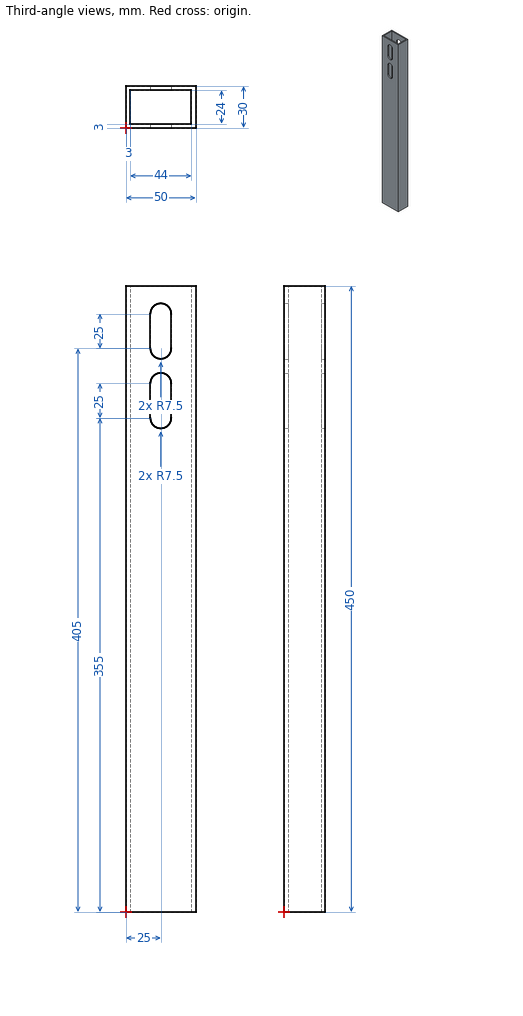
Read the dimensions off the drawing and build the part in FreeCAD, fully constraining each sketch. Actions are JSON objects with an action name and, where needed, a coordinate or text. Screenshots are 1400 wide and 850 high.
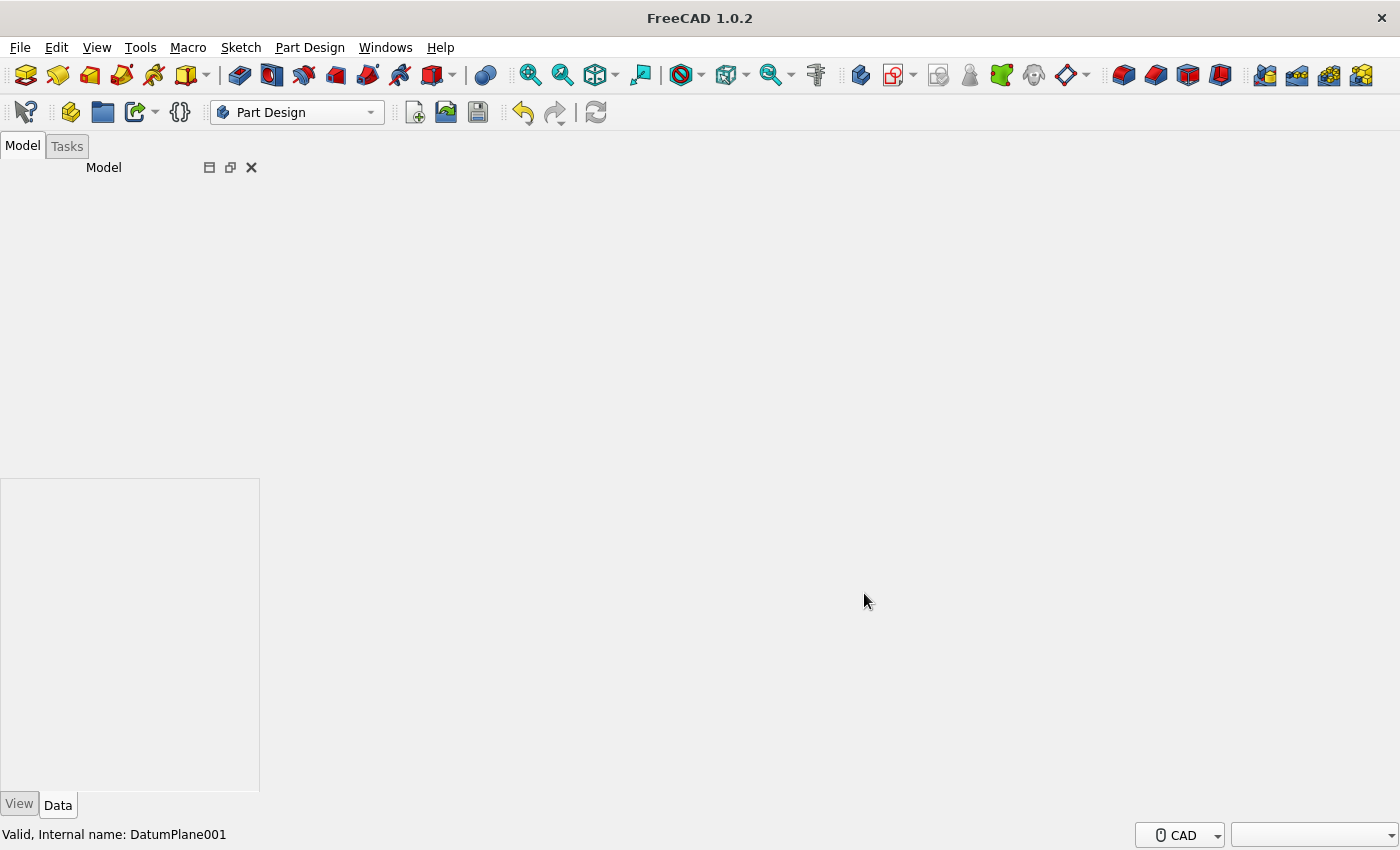
{"action": "left_click", "coordinate": [414, 112]}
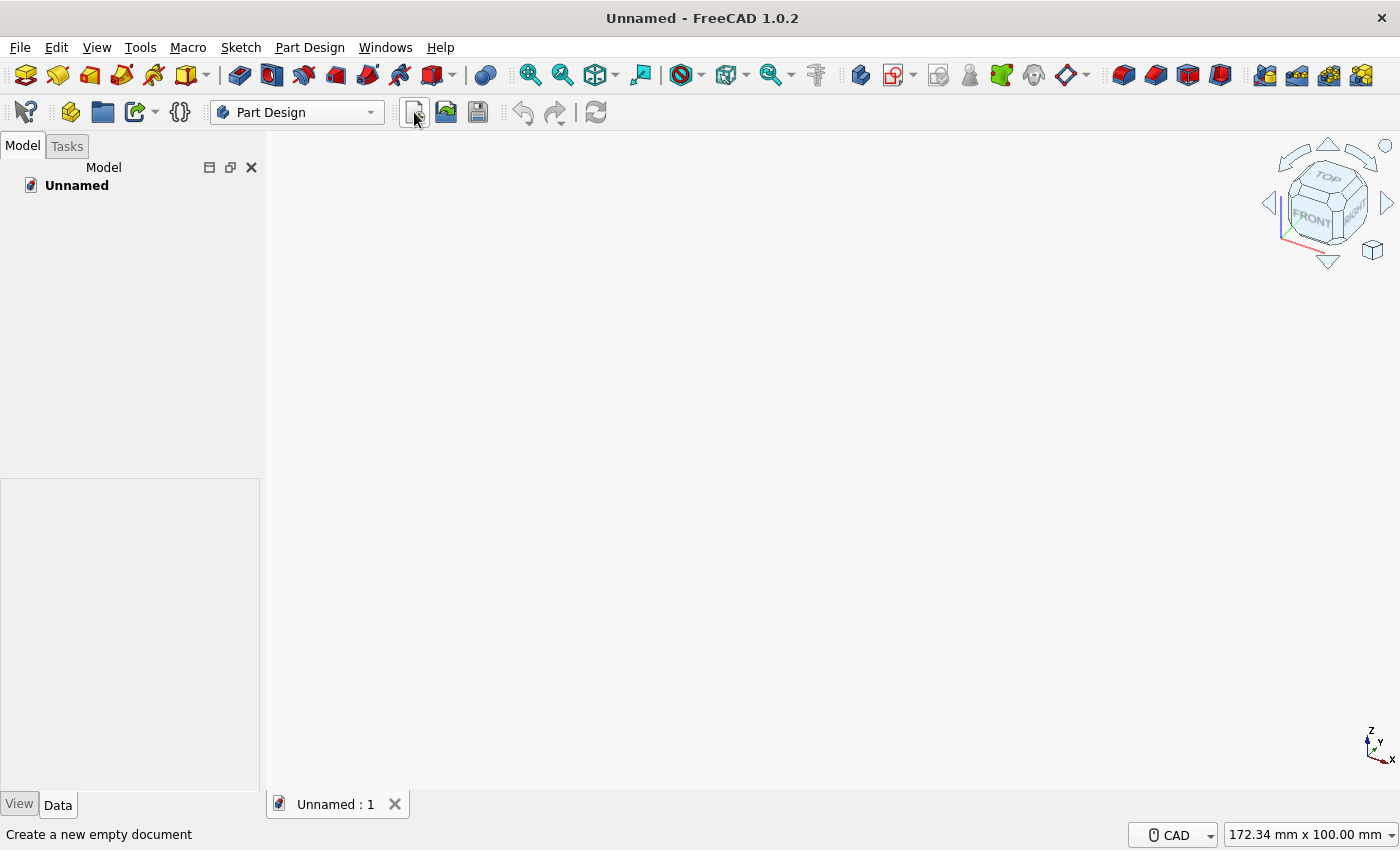
{"action": "left_click", "coordinate": [894, 76]}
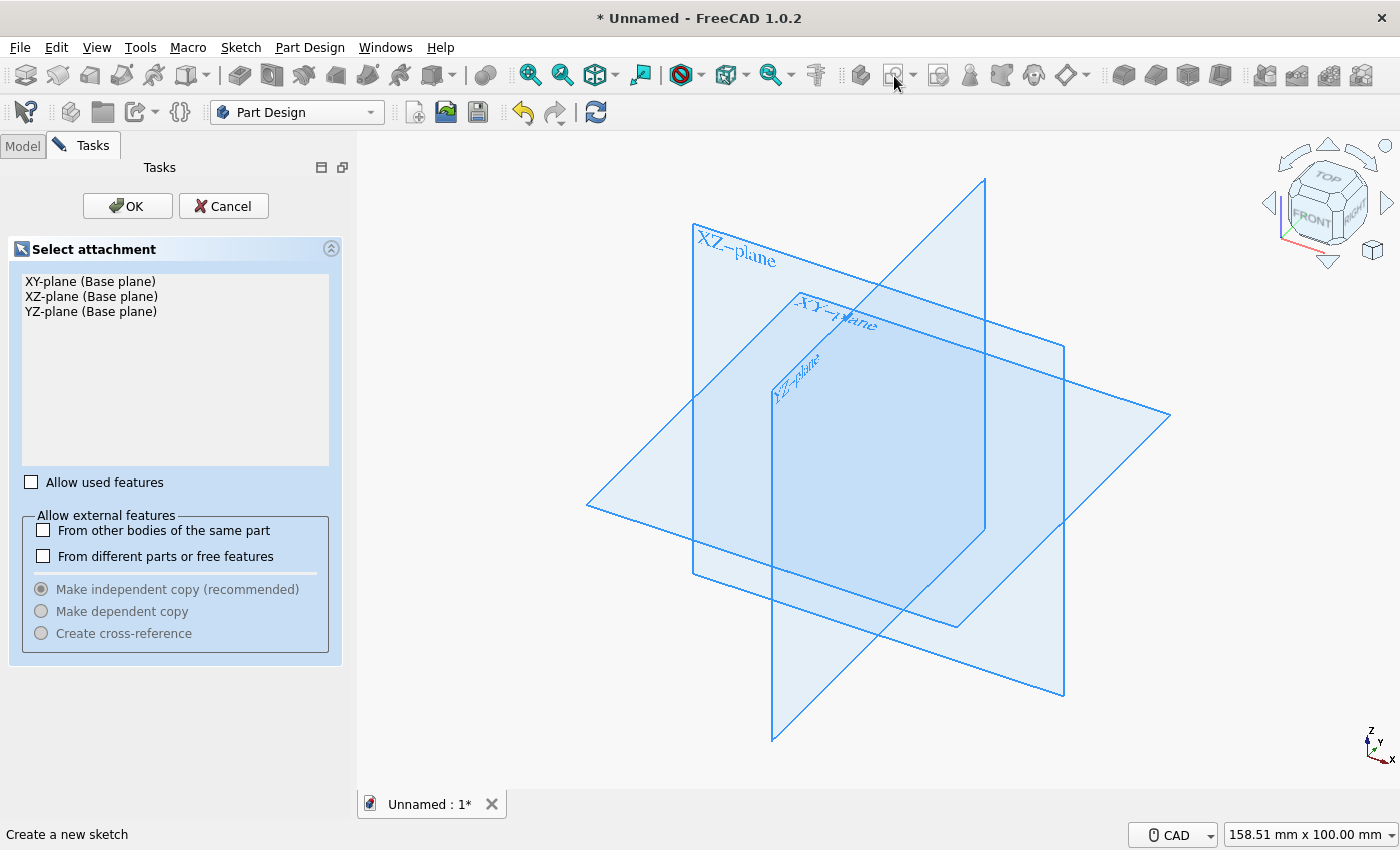
{"action": "left_click", "coordinate": [82, 282]}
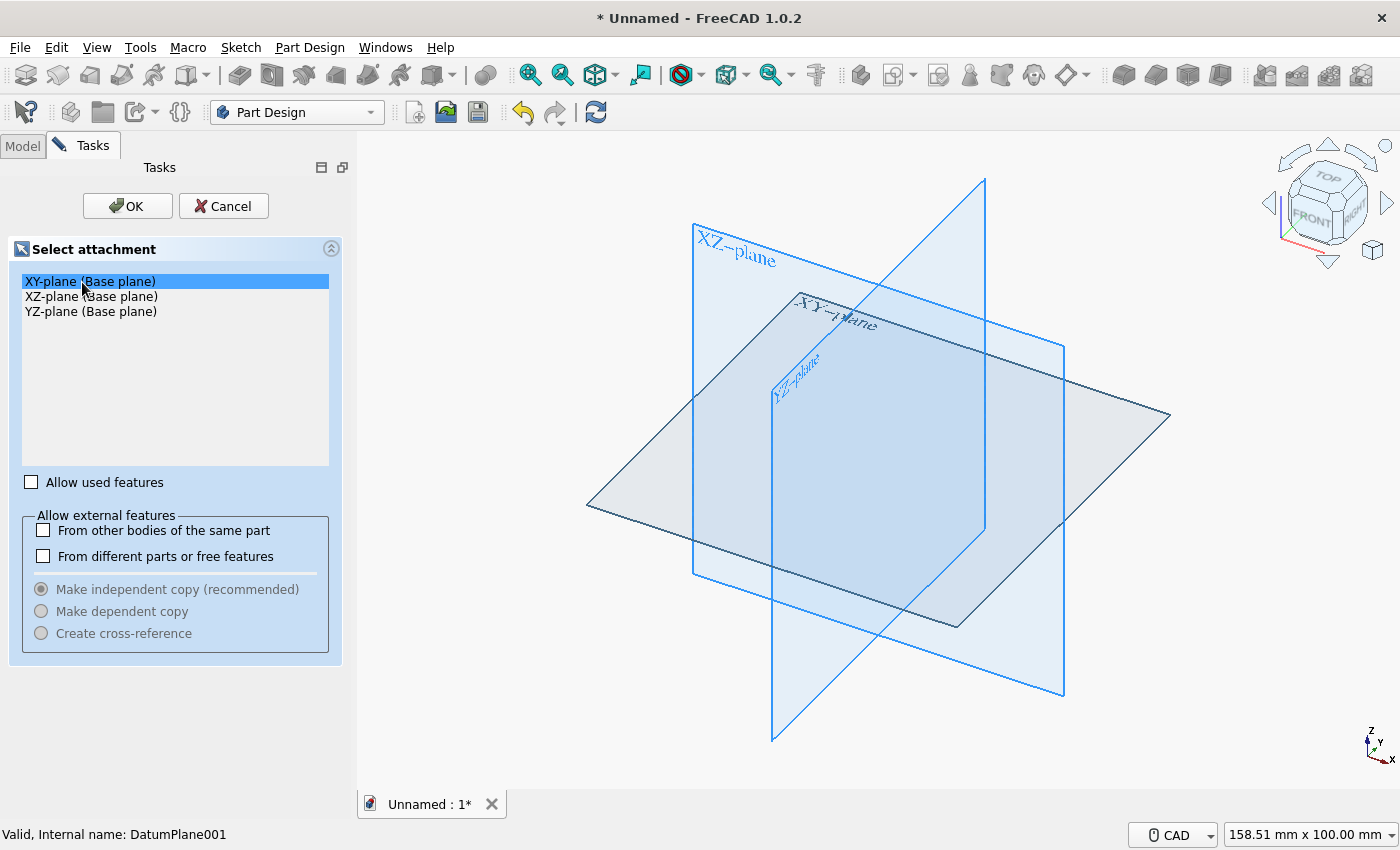
{"action": "left_click", "coordinate": [128, 206]}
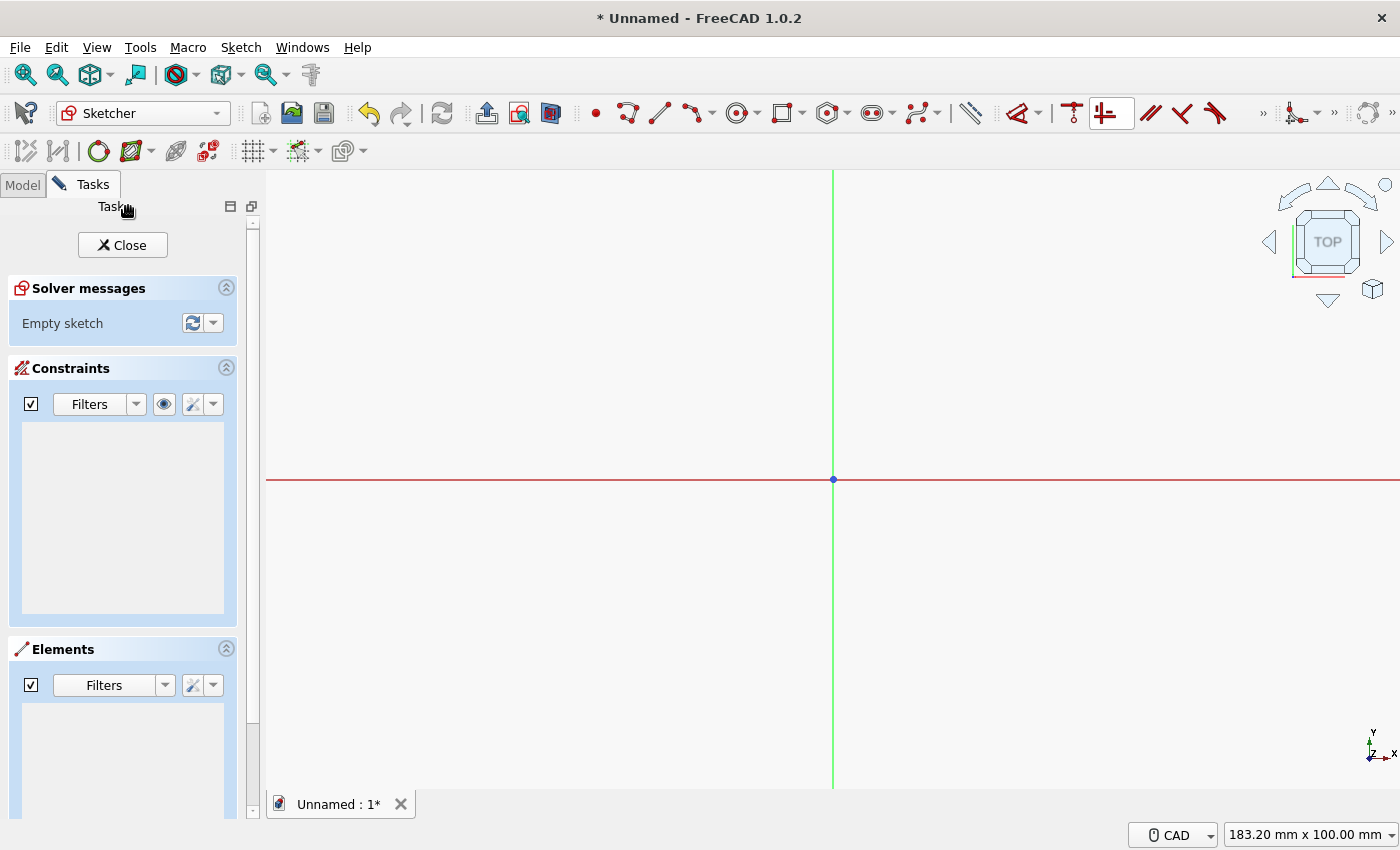
{"action": "scroll", "coordinate": [1170, 311], "scroll_direction": "up", "scroll_amount": 4}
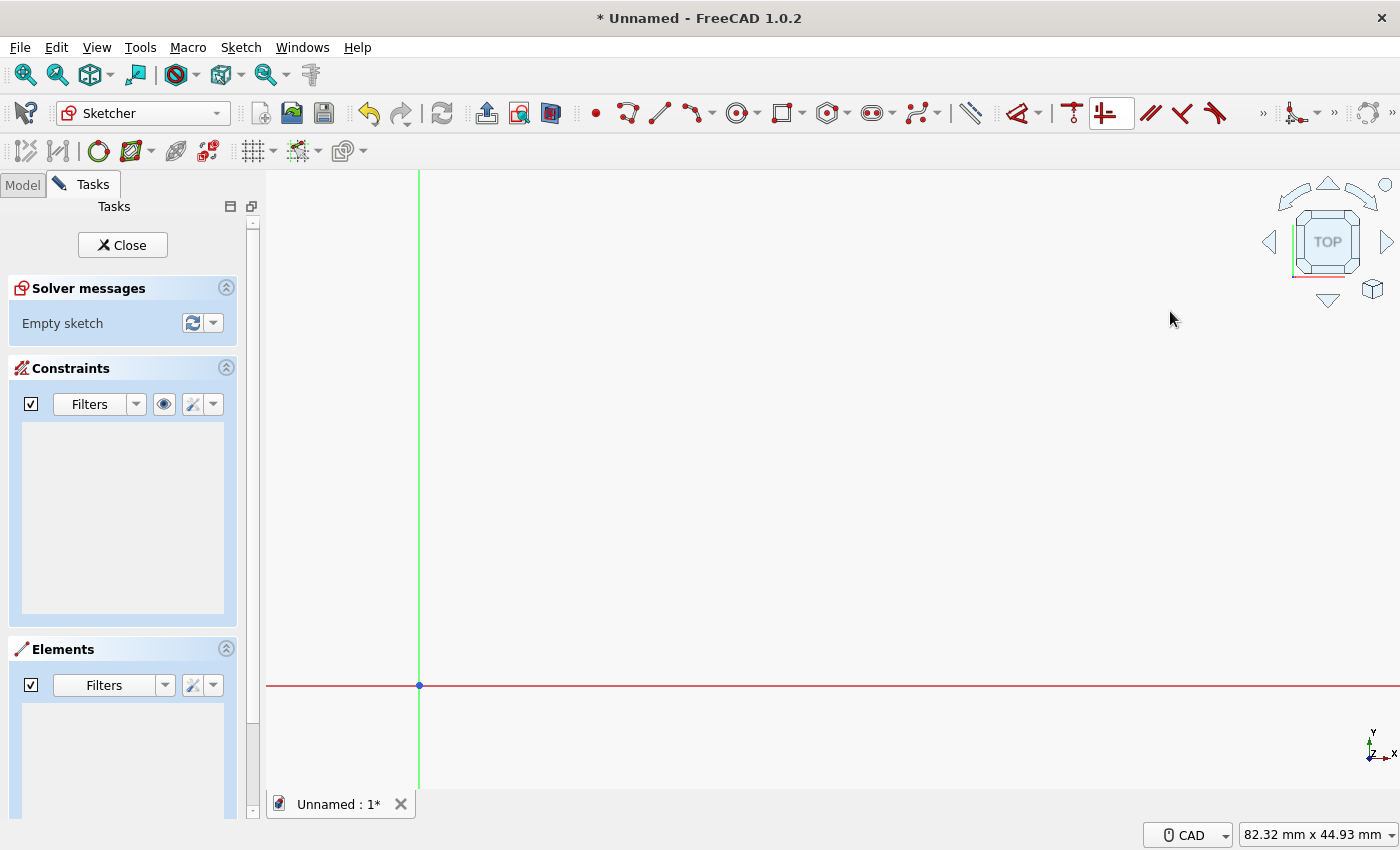
{"action": "left_click", "coordinate": [782, 114]}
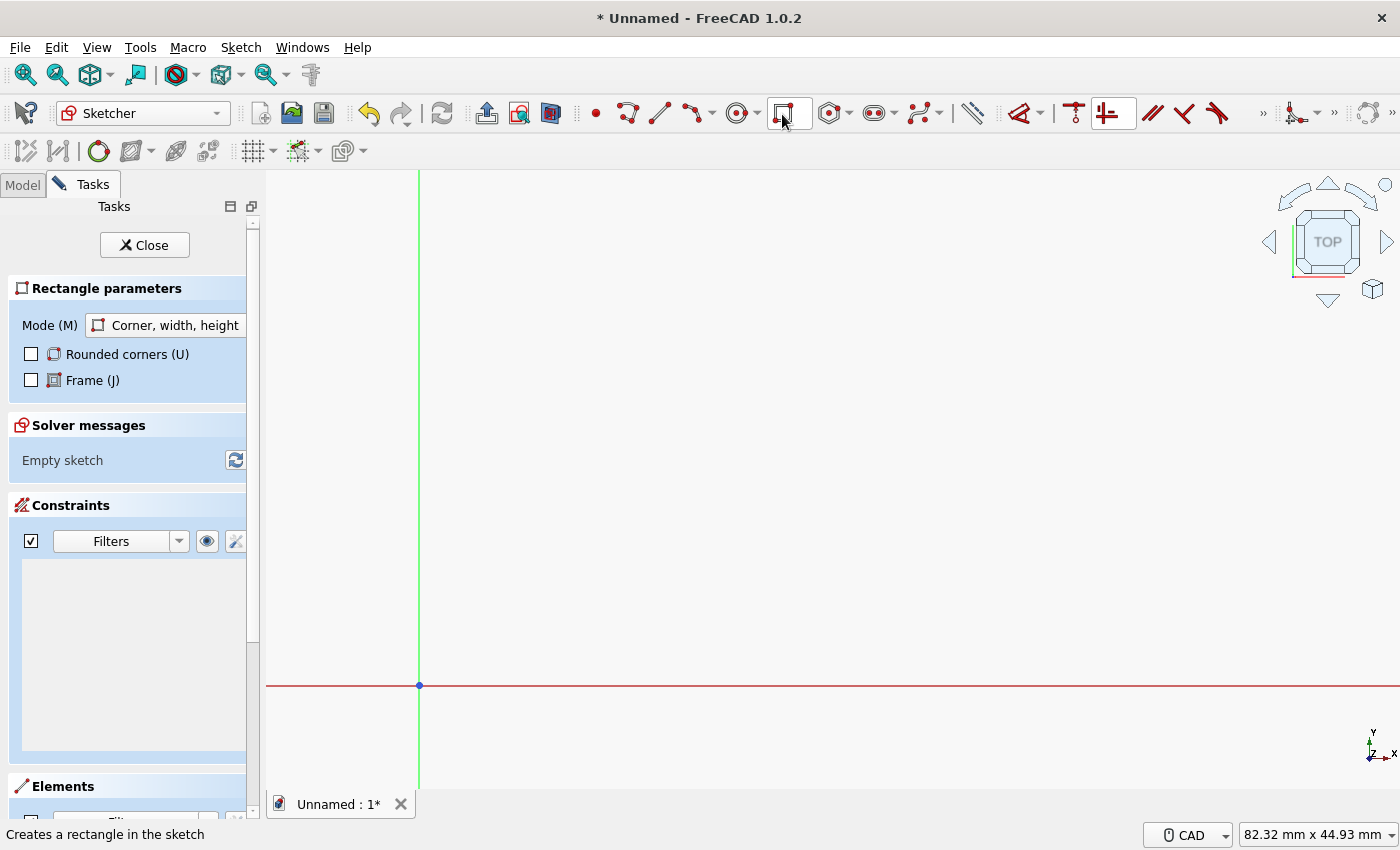
{"action": "left_click", "coordinate": [419, 686]}
{"action": "mouse_move", "coordinate": [1108, 272]}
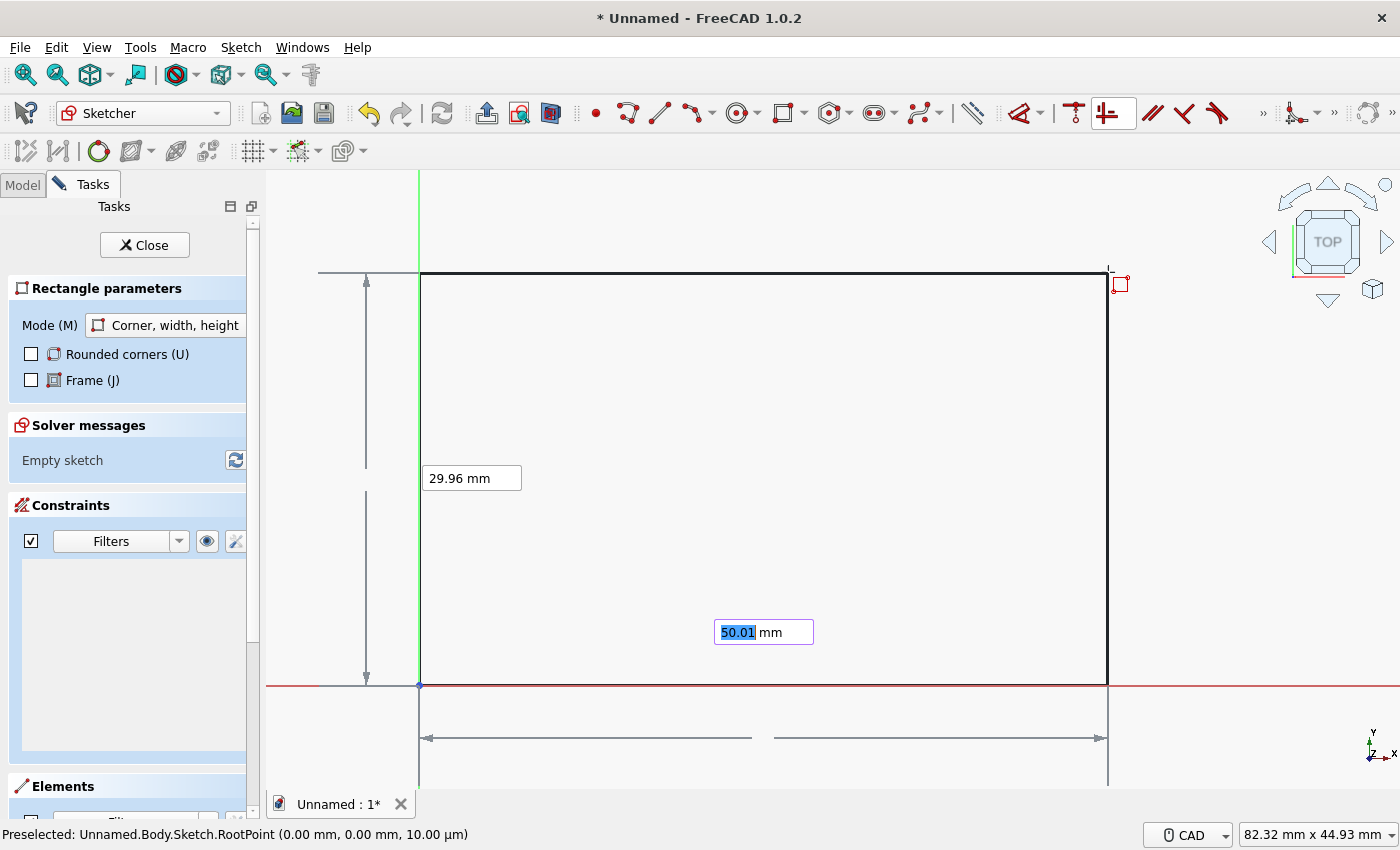
{"action": "type", "text": "50"}
{"action": "key", "text": "Tab"}
{"action": "type", "text": "30"}
{"action": "key", "text": "Return"}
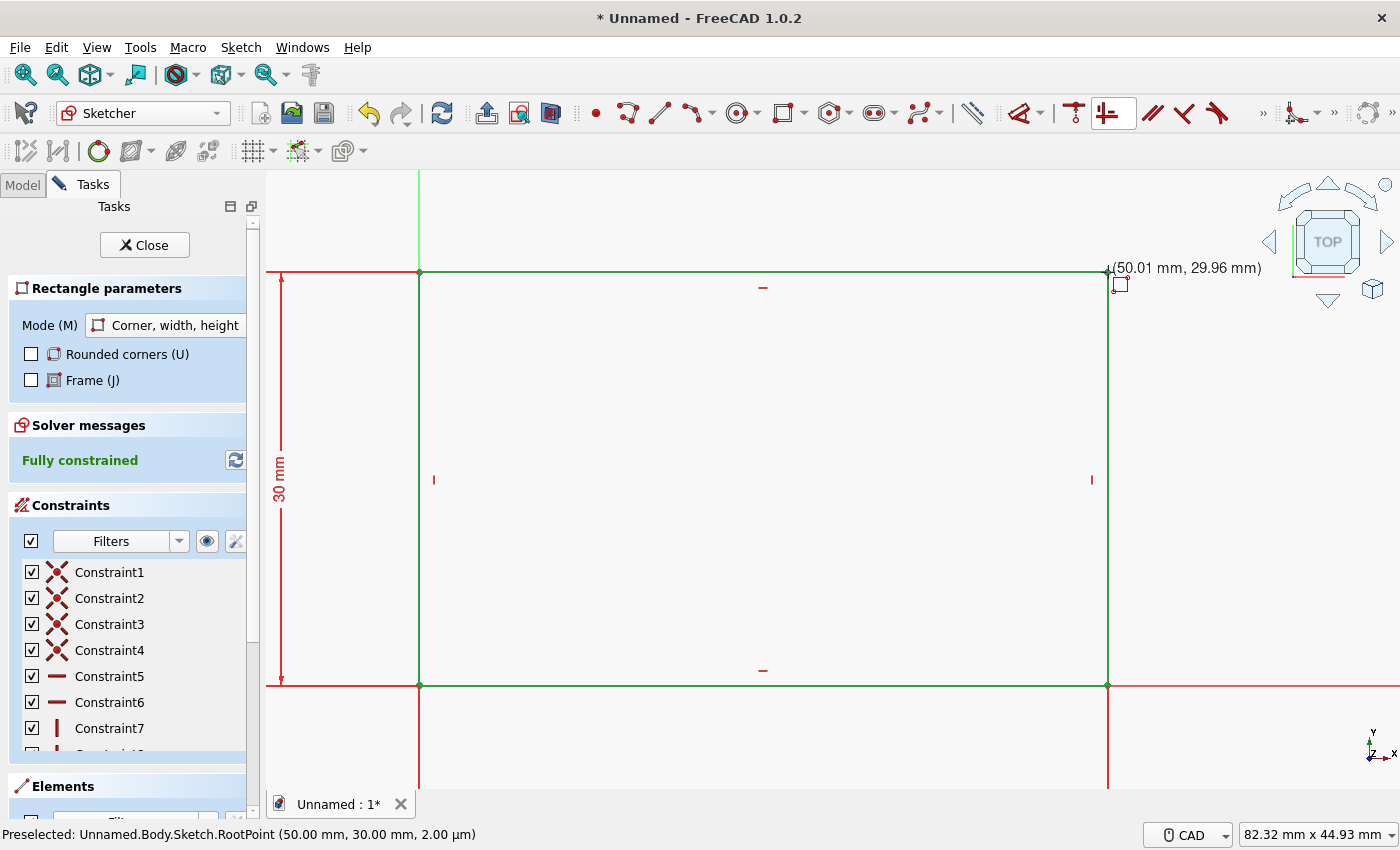
{"action": "left_click", "coordinate": [460, 314]}
{"action": "mouse_move", "coordinate": [1066, 644]}